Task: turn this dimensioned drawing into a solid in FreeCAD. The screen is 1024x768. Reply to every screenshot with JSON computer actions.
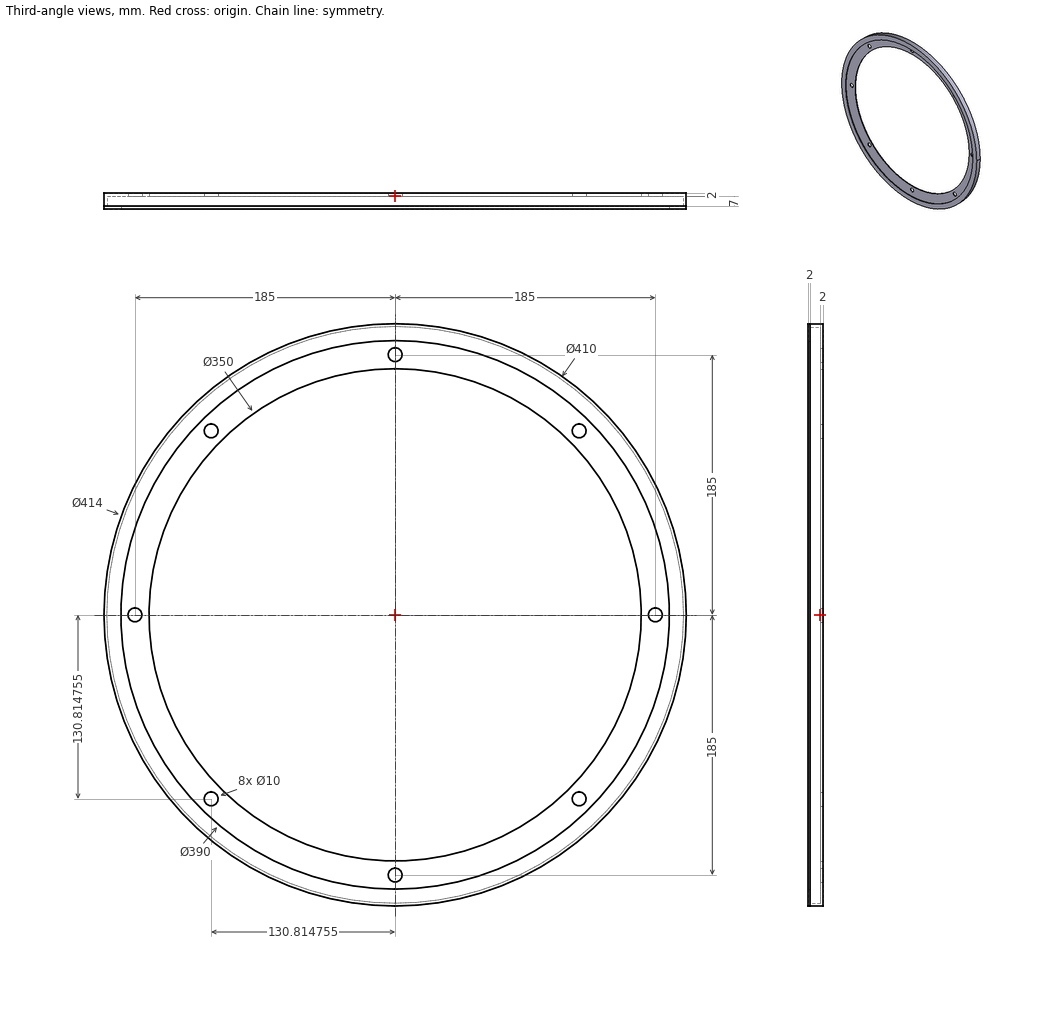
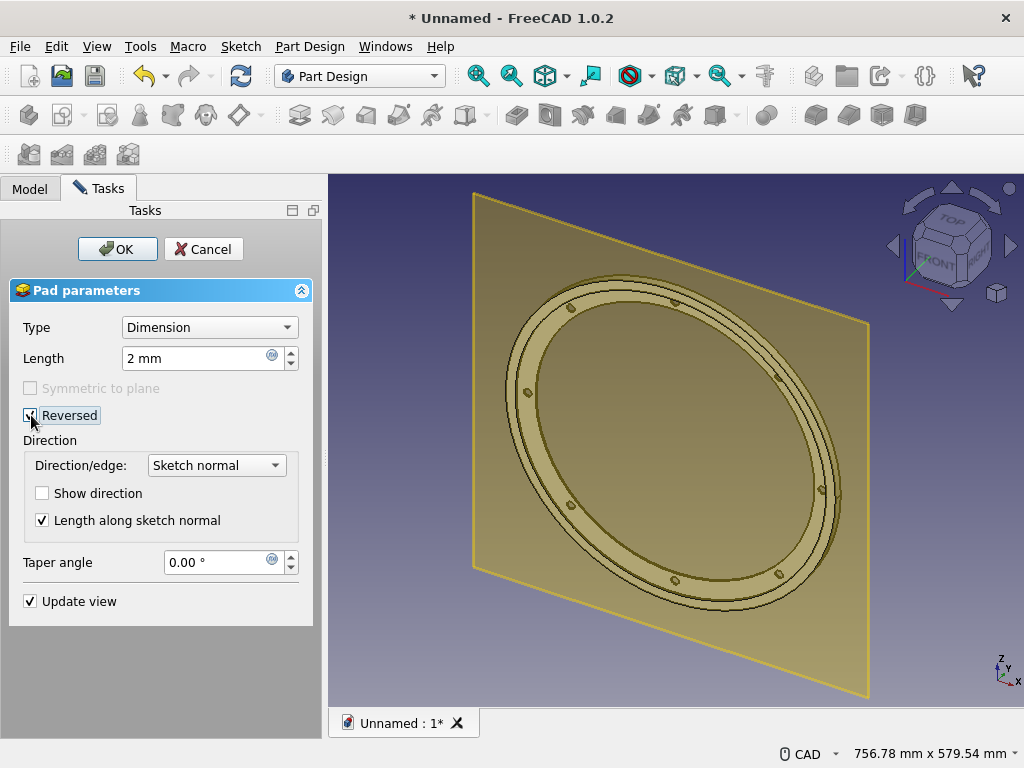
{"action": "left_click", "coordinate": [118, 249]}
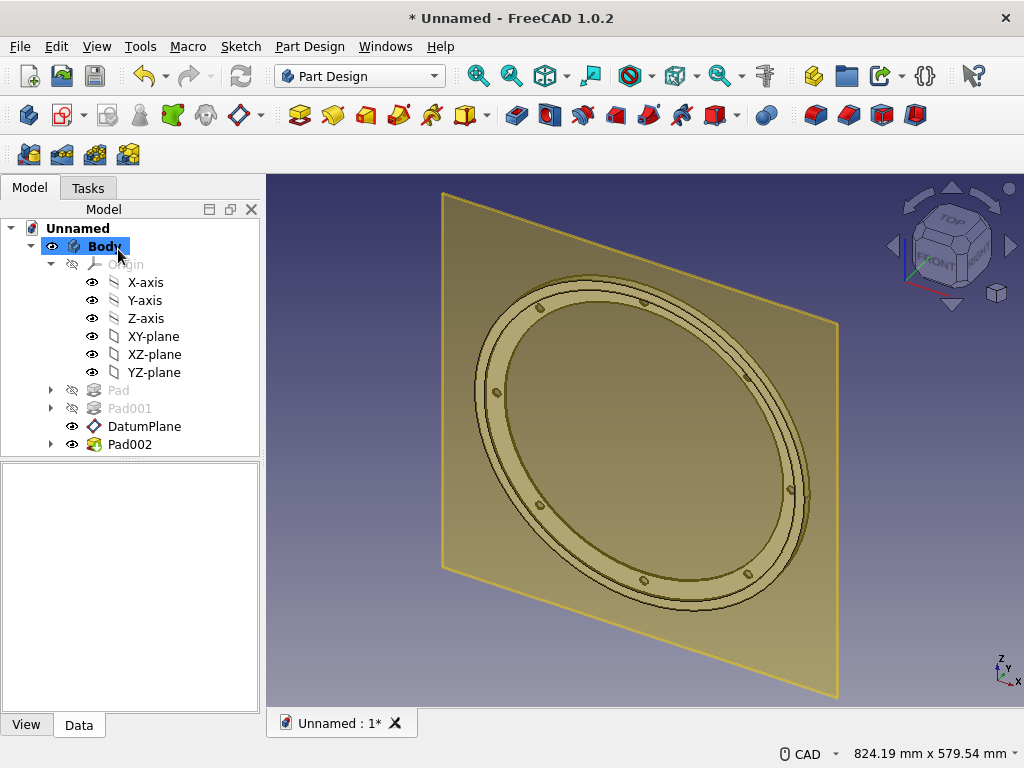
{"action": "left_click", "coordinate": [117, 426]}
{"action": "key", "text": "space"}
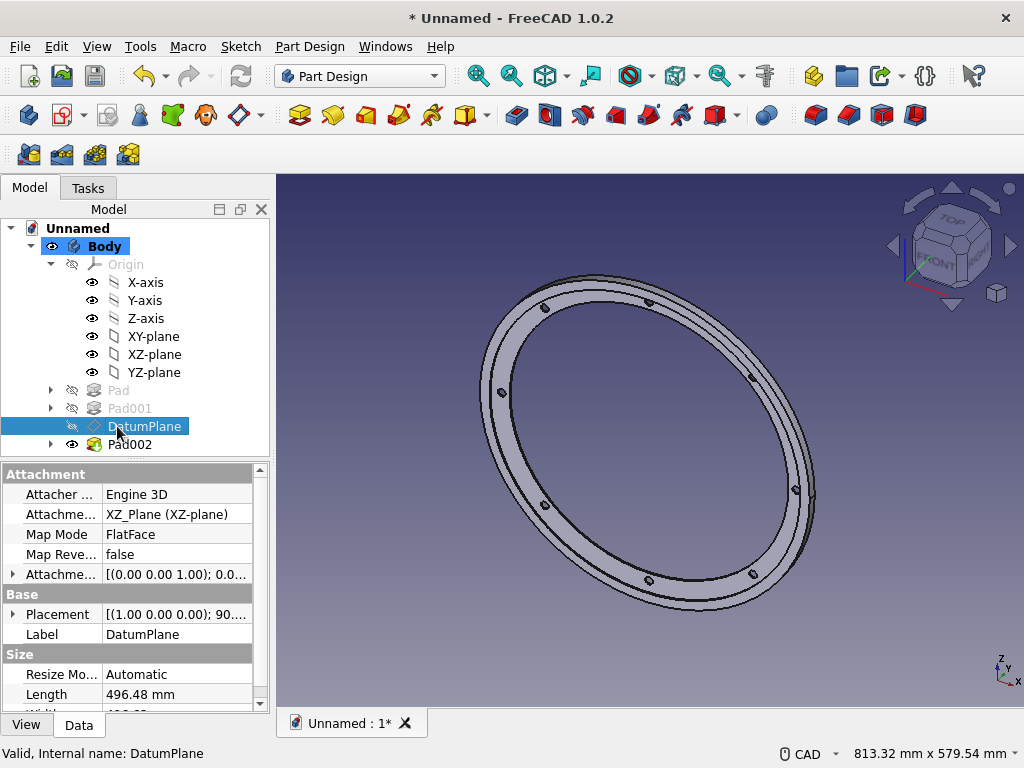
{"action": "key", "text": "0"}